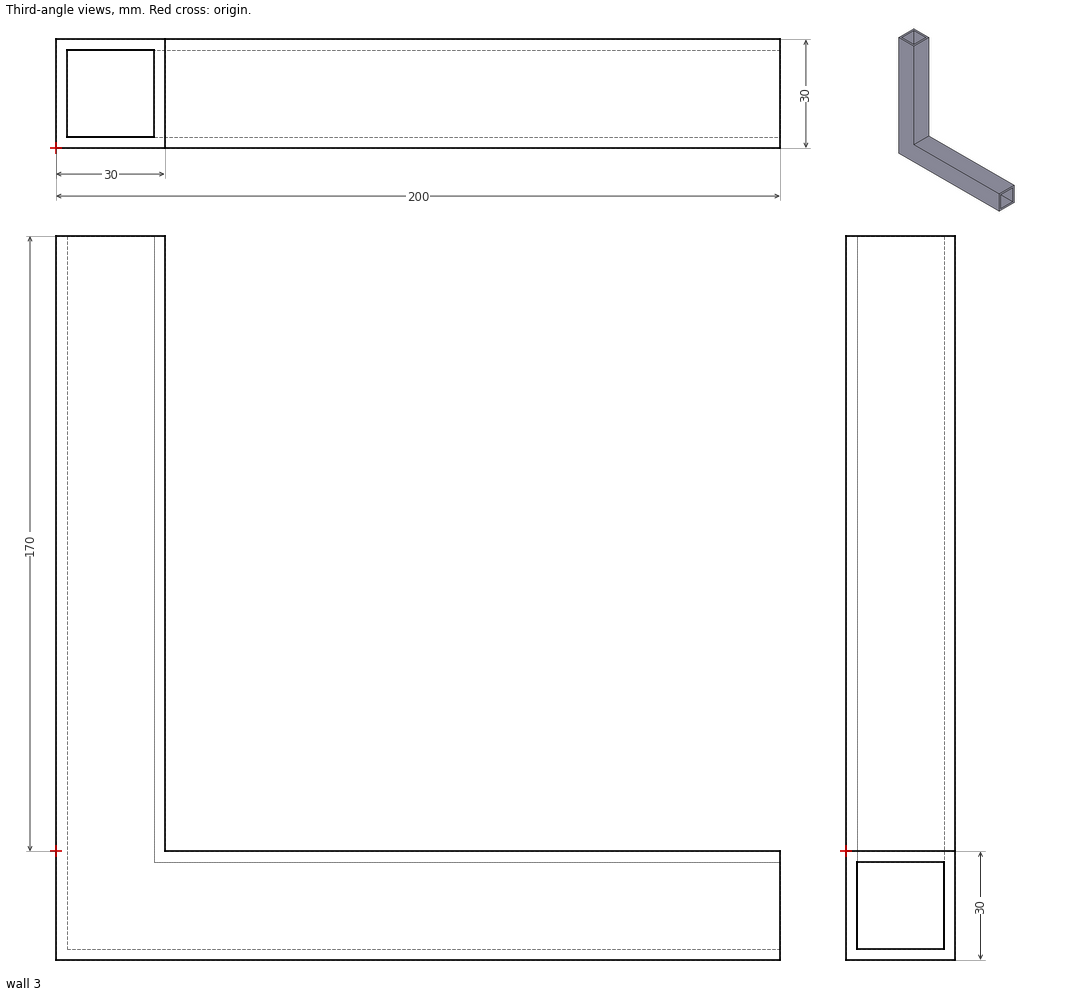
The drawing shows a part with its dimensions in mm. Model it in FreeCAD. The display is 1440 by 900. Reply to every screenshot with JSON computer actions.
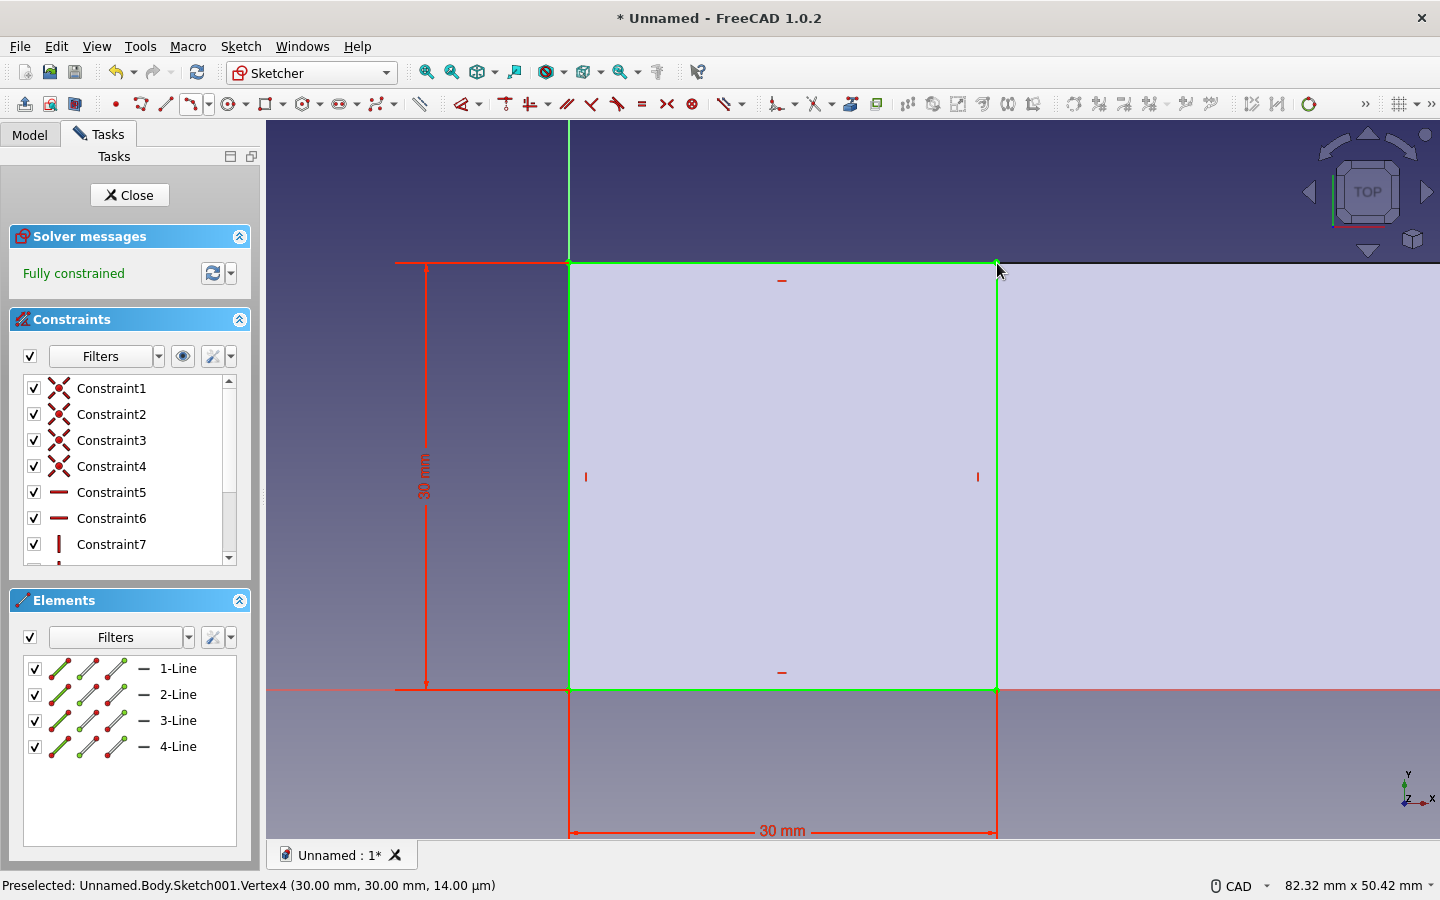
{"action": "left_click", "coordinate": [130, 195]}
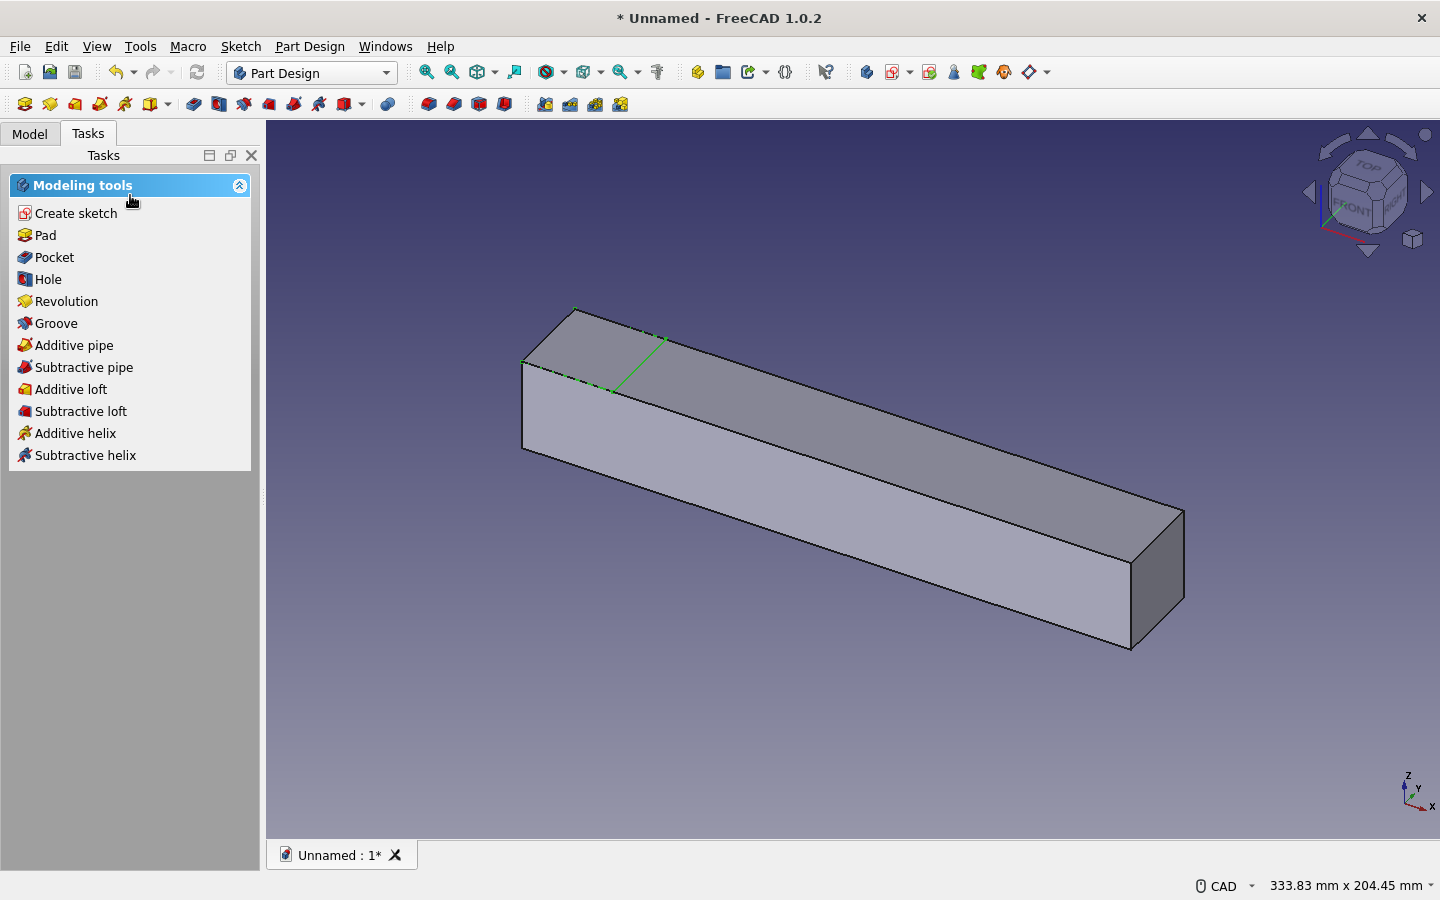
{"action": "left_click", "coordinate": [25, 104]}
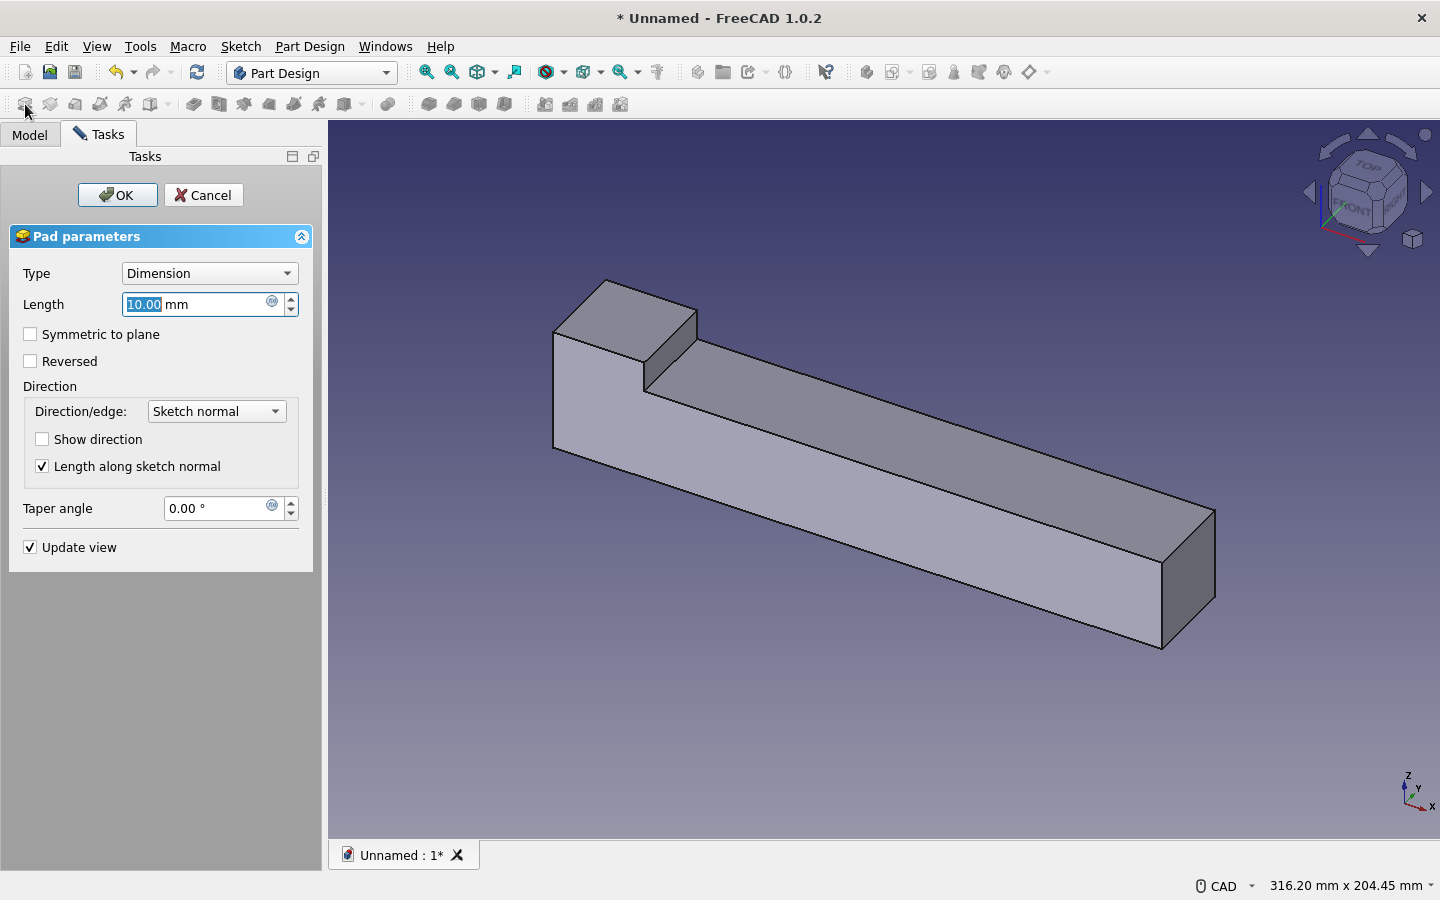
{"action": "type", "text": "170"}
{"action": "key", "text": "Tab"}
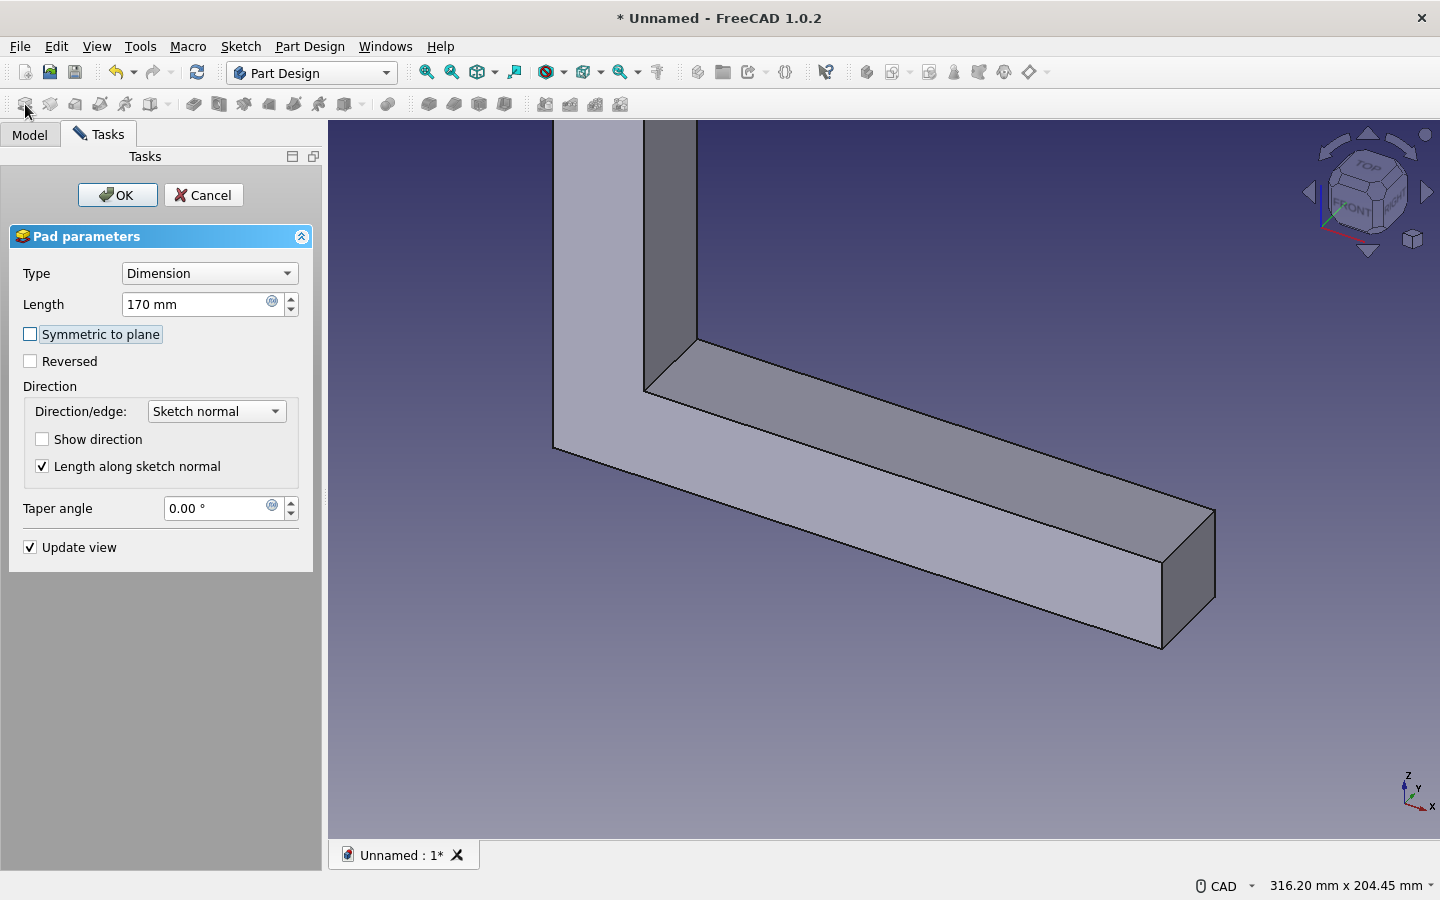
{"action": "left_click", "coordinate": [118, 195]}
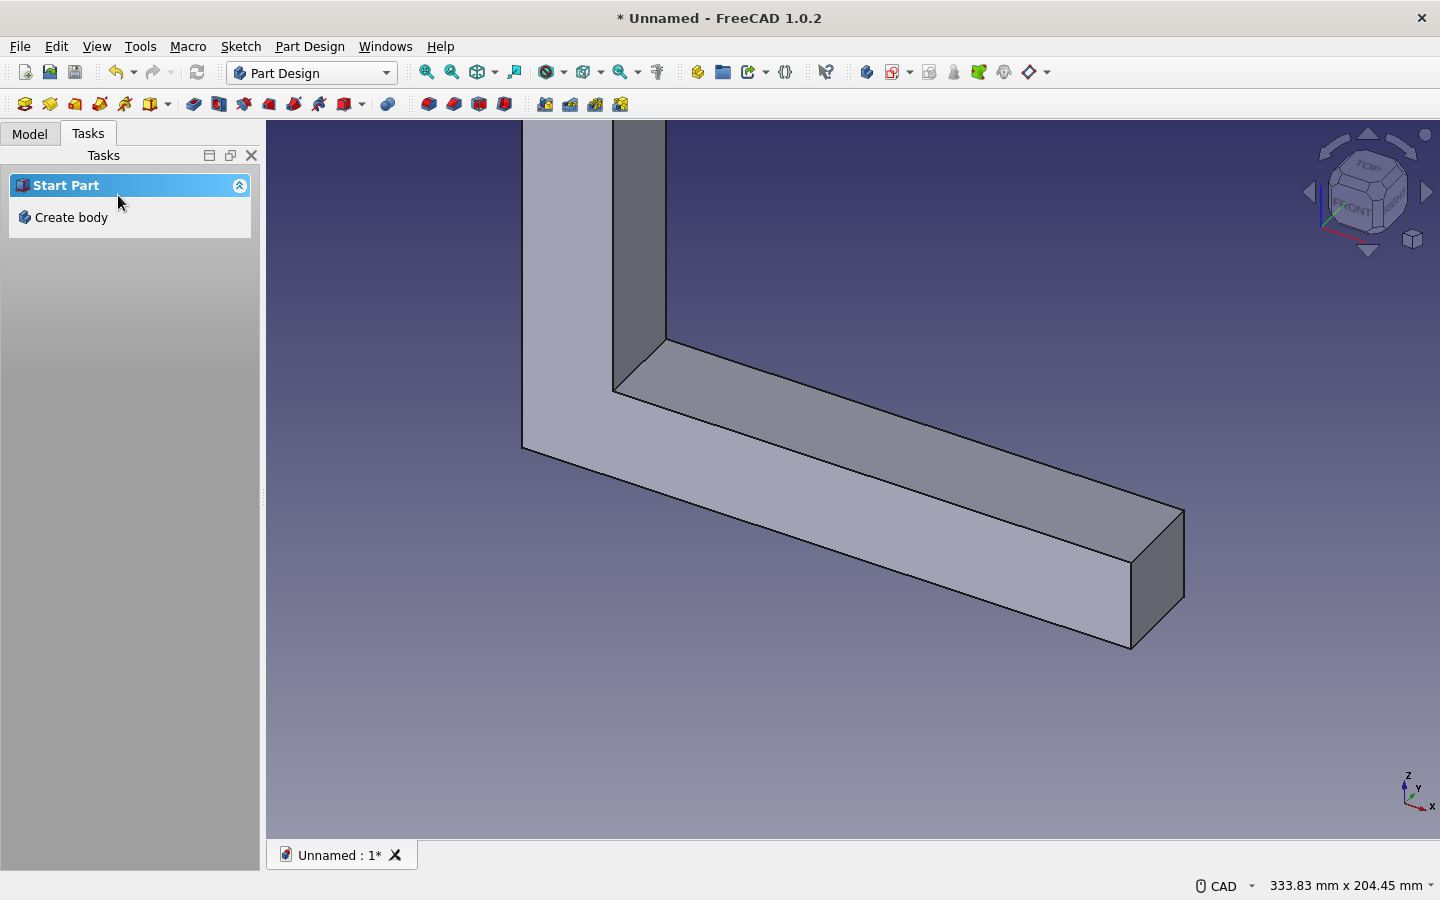
{"action": "left_click", "coordinate": [427, 72]}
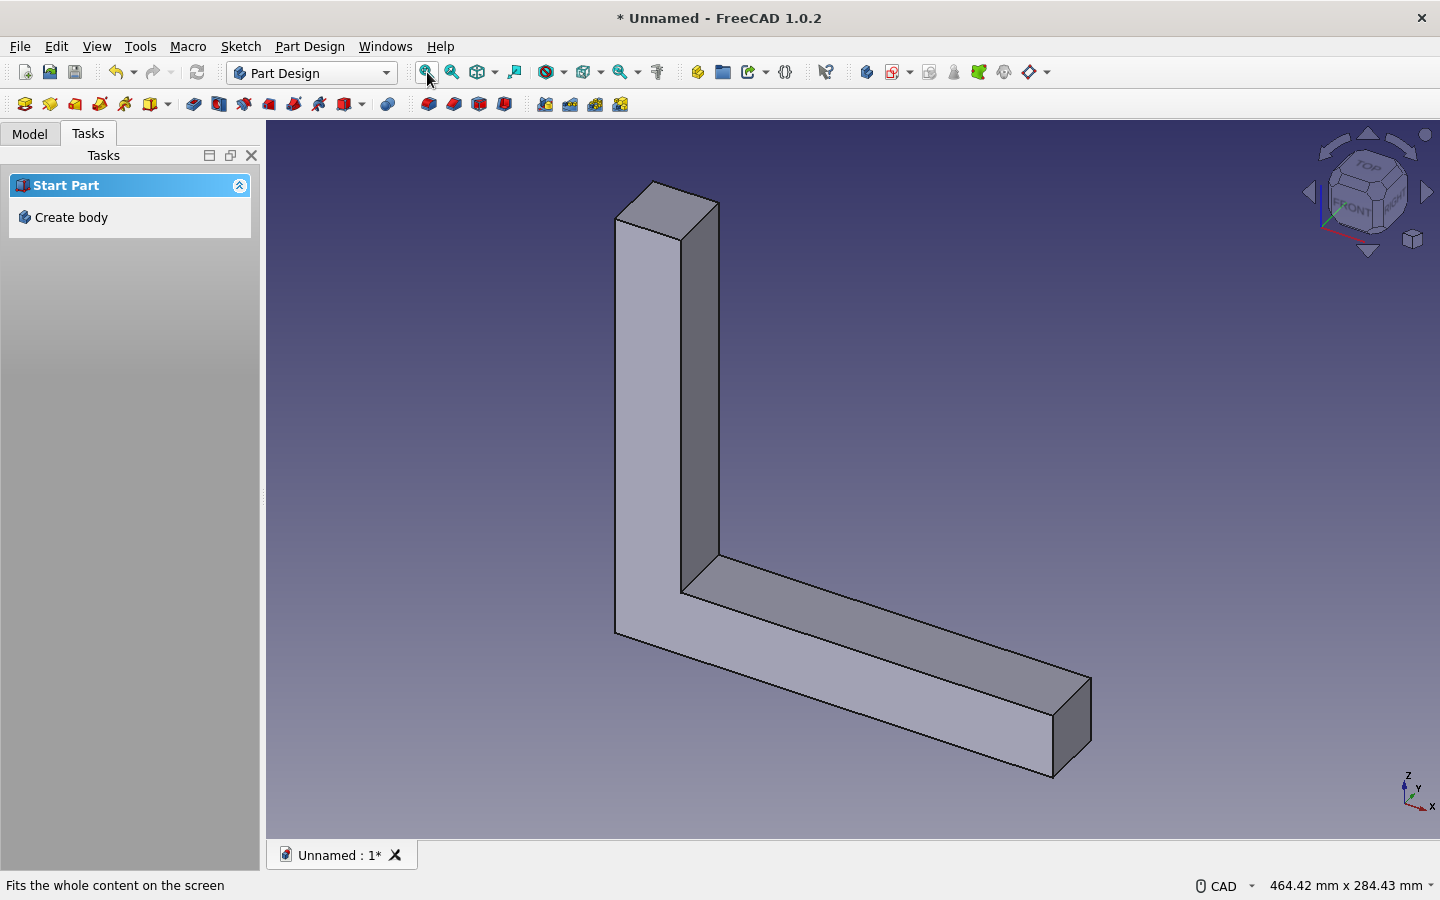
{"action": "left_click", "coordinate": [667, 210]}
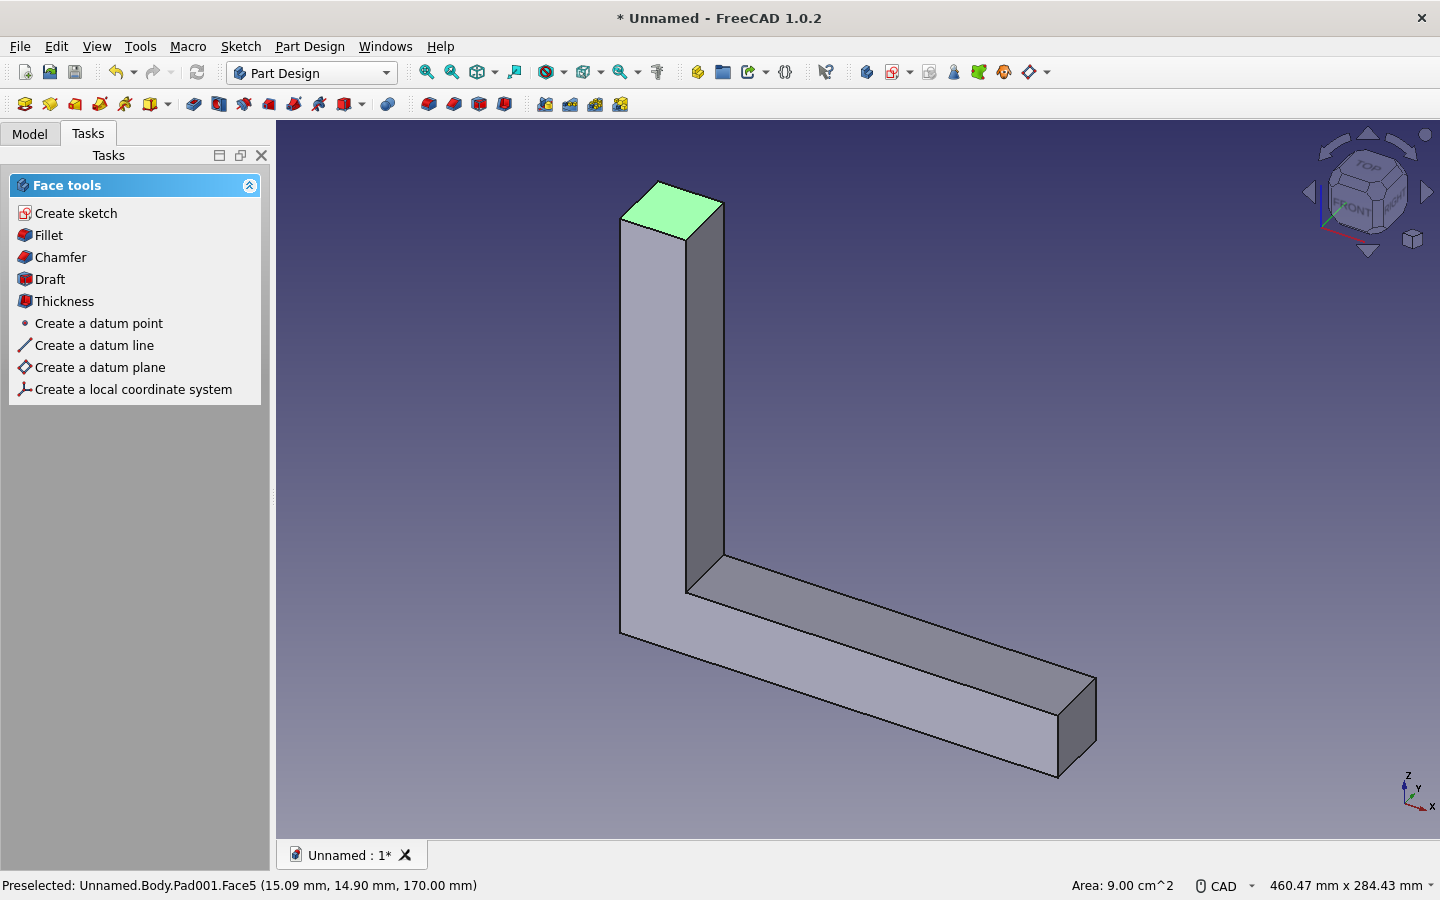
{"action": "left_click", "coordinate": [1077, 727], "text": "ctrl"}